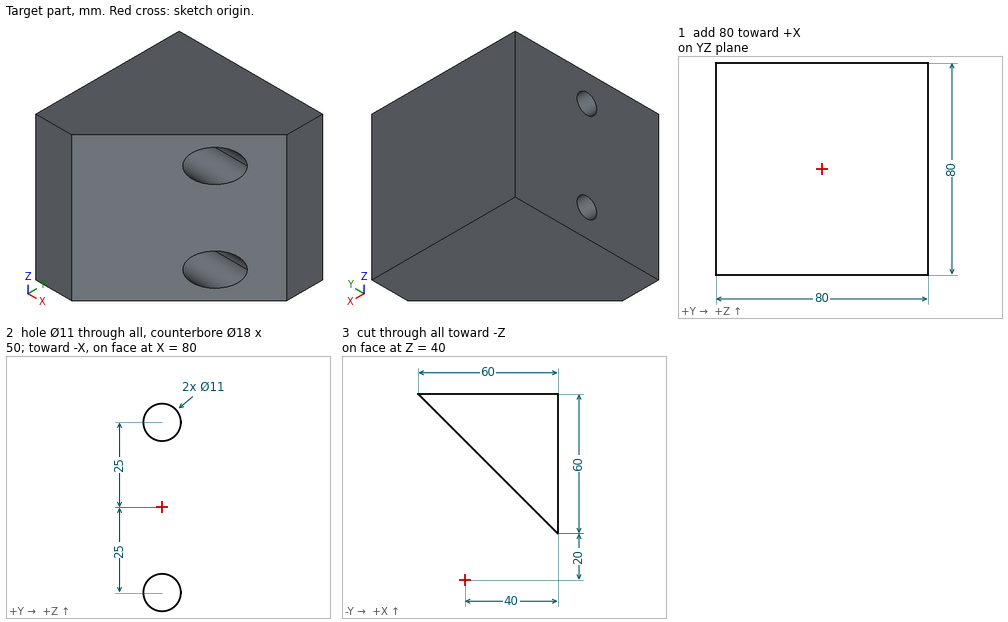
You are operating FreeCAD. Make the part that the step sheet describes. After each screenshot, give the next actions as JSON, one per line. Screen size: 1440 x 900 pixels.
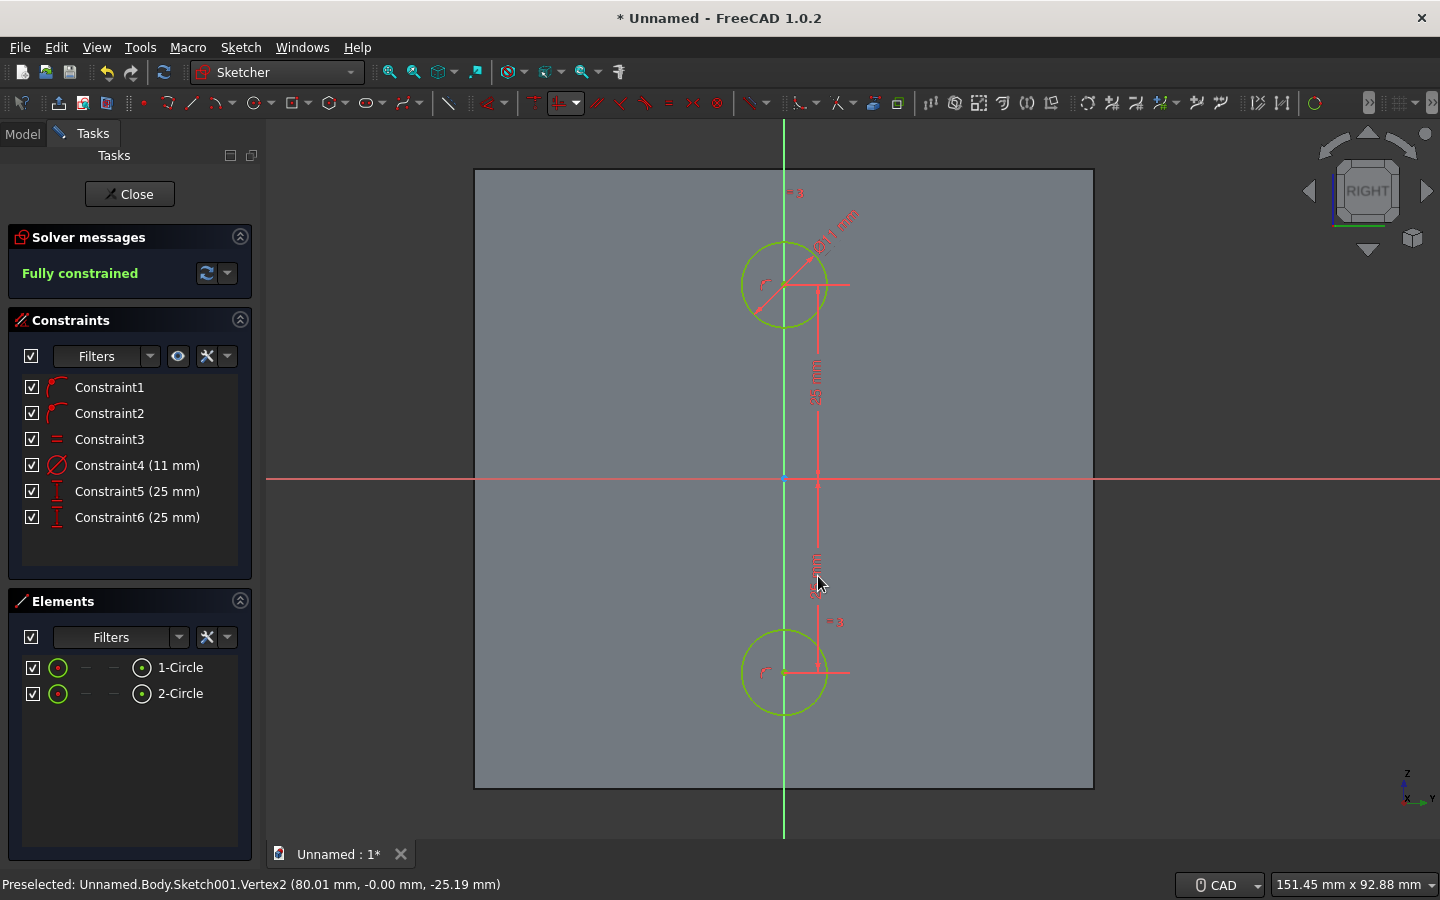
{"action": "left_click", "coordinate": [130, 194]}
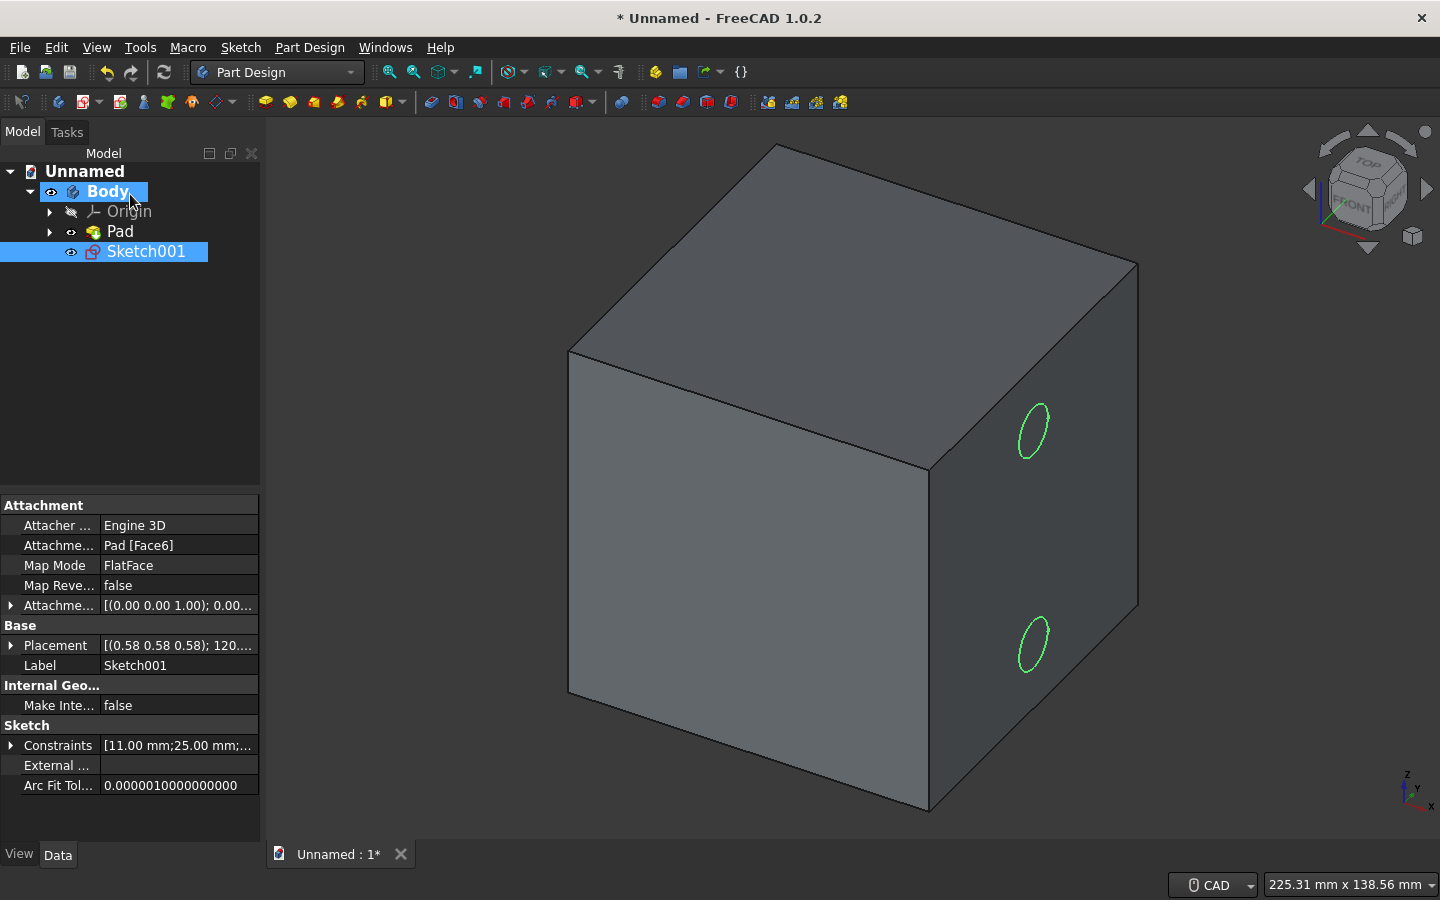
{"action": "left_click", "coordinate": [456, 102]}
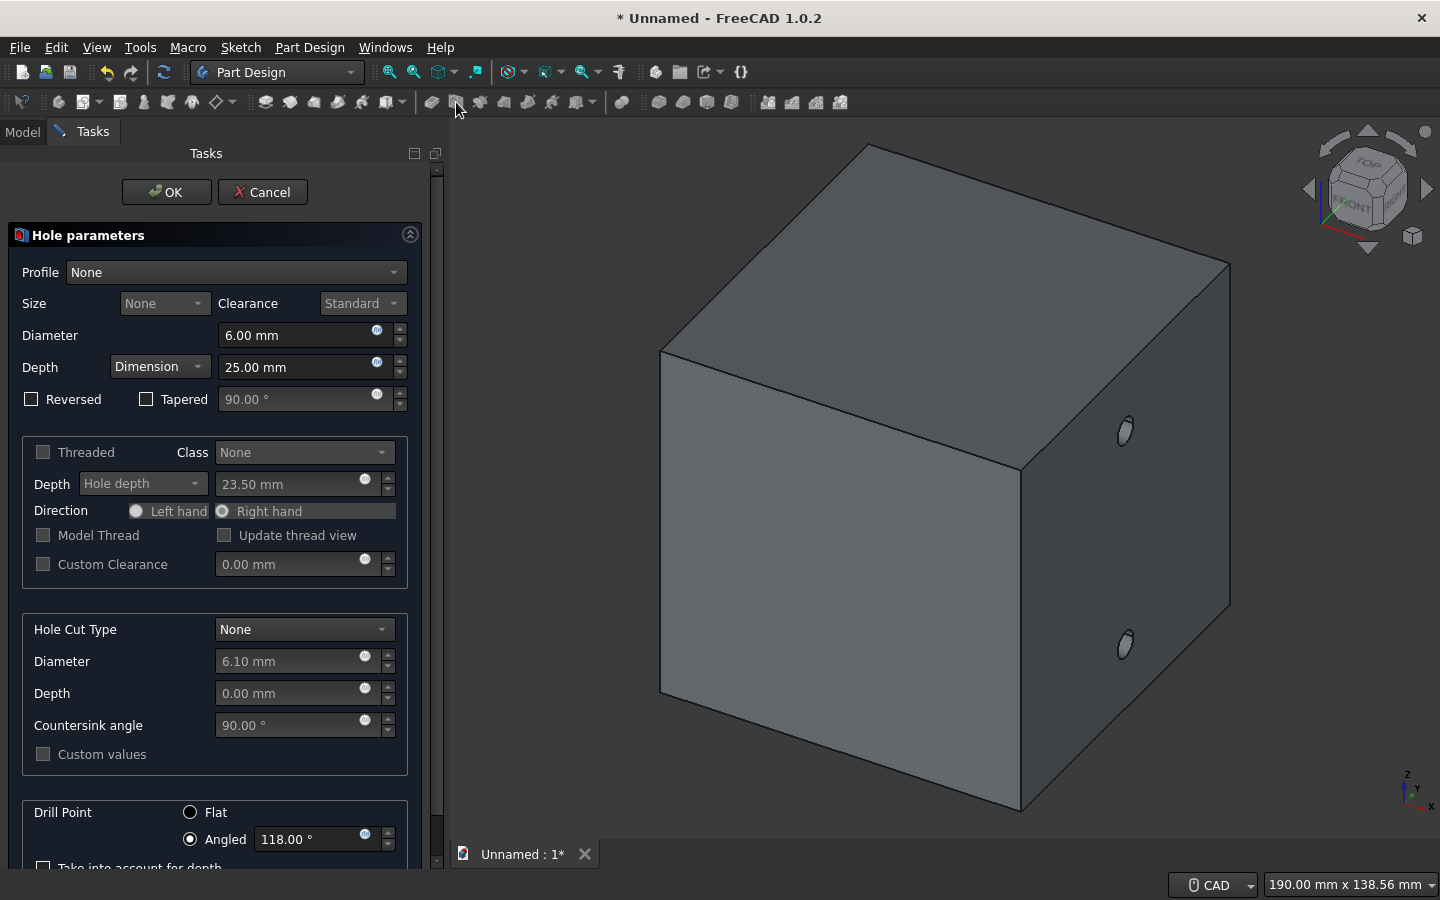
{"action": "triple_click", "coordinate": [305, 335]}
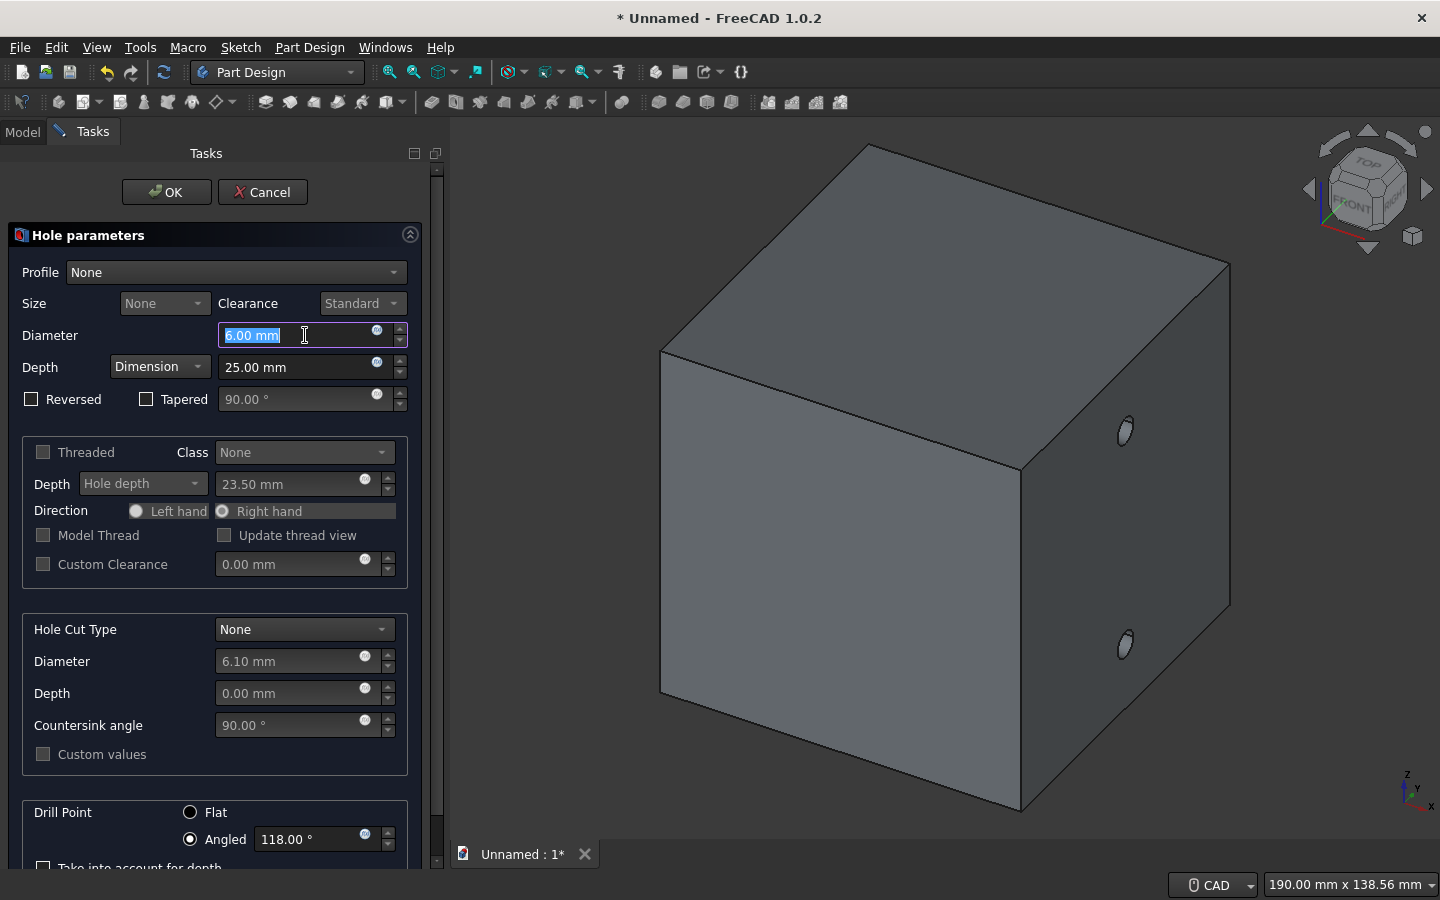
{"action": "type", "text": "11"}
{"action": "key", "text": "Tab"}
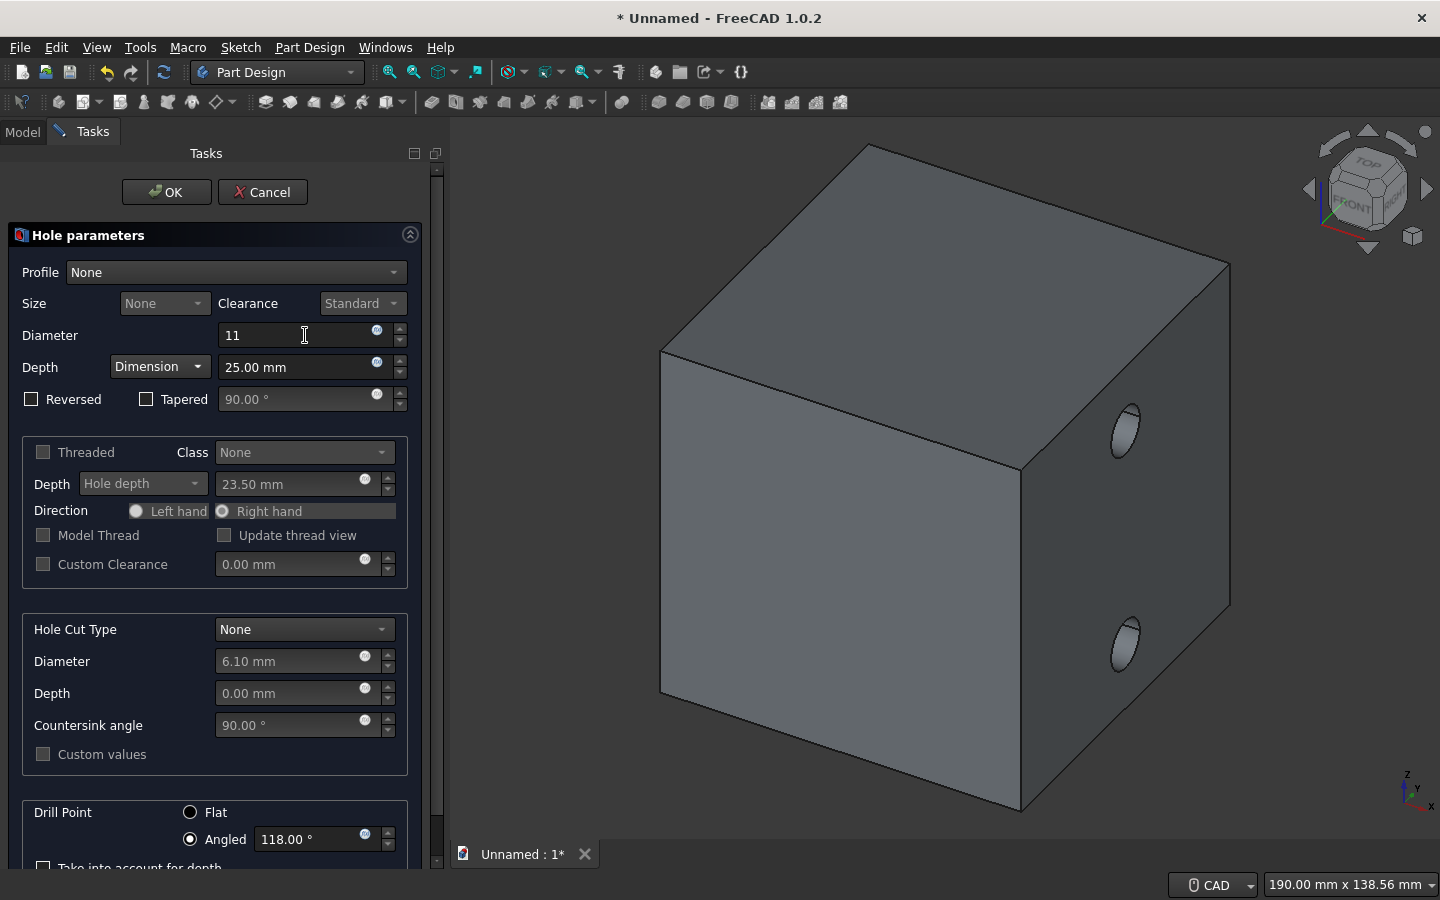
{"action": "left_click", "coordinate": [161, 366]}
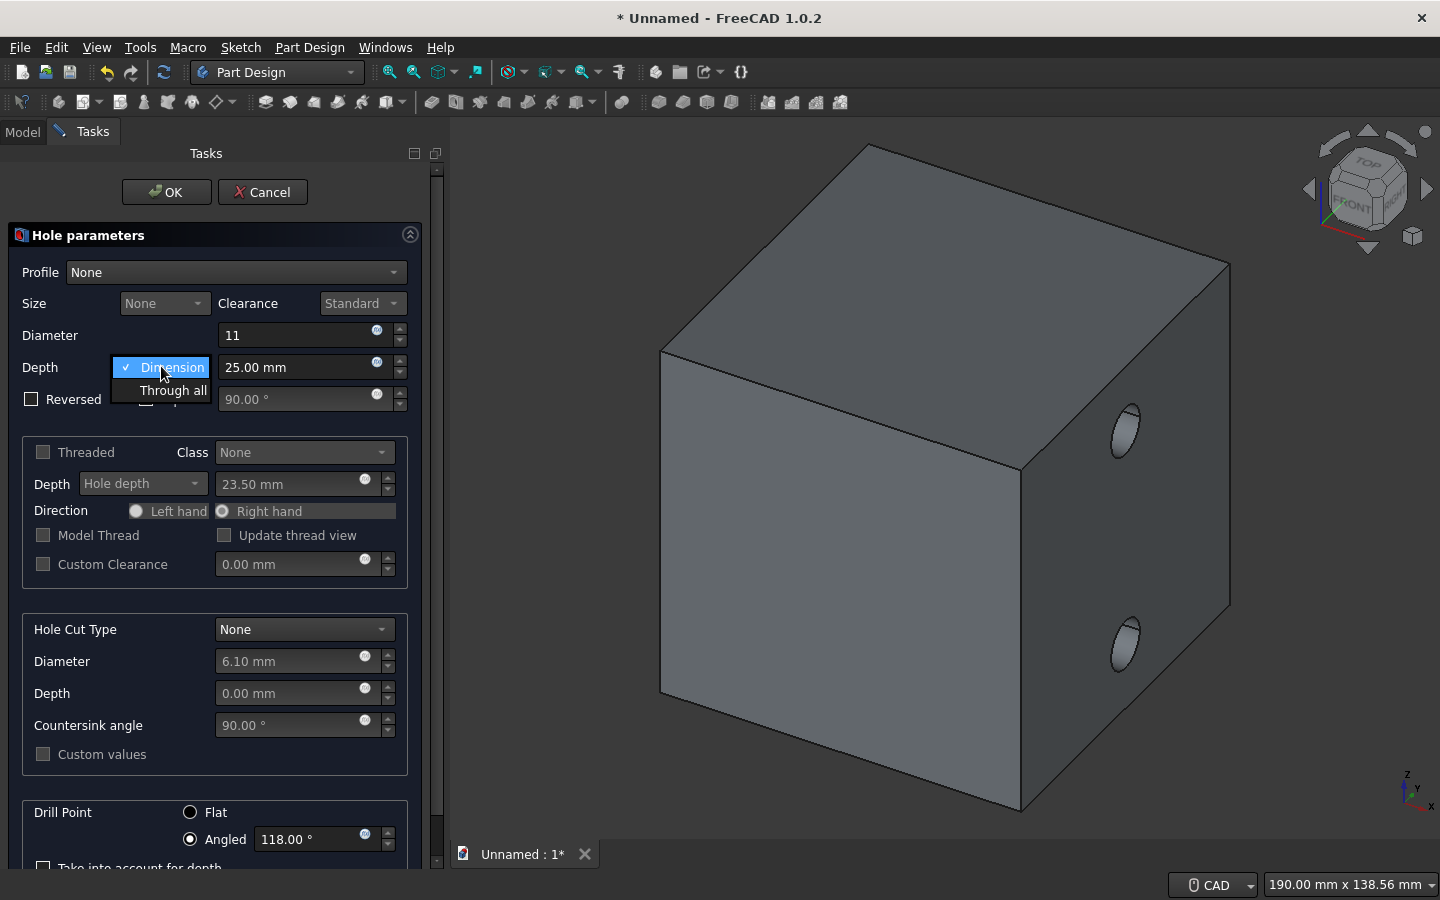
{"action": "left_click", "coordinate": [160, 390]}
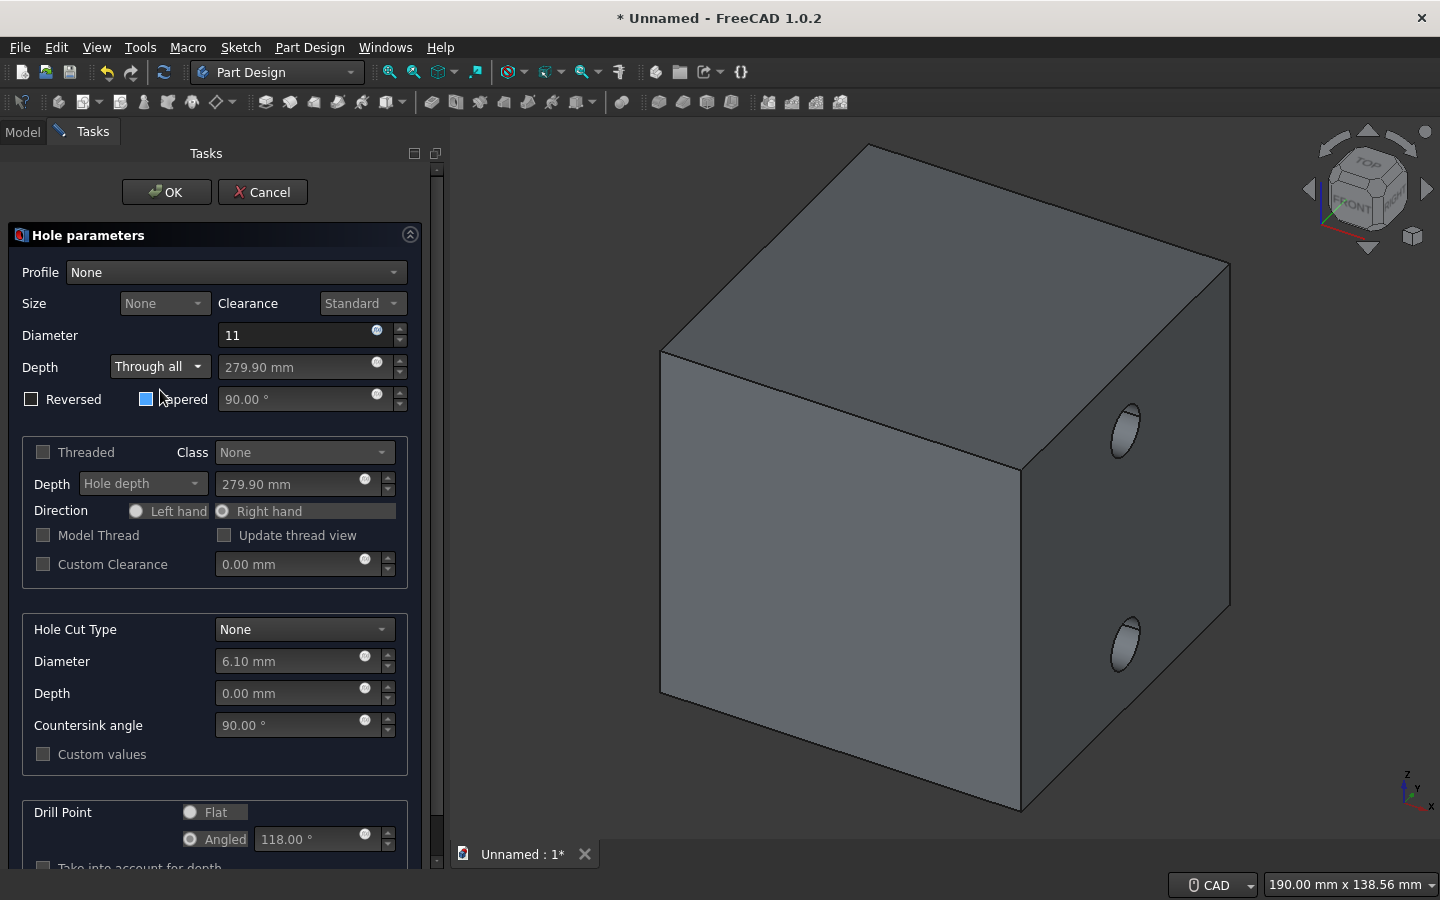
{"action": "left_click", "coordinate": [306, 630]}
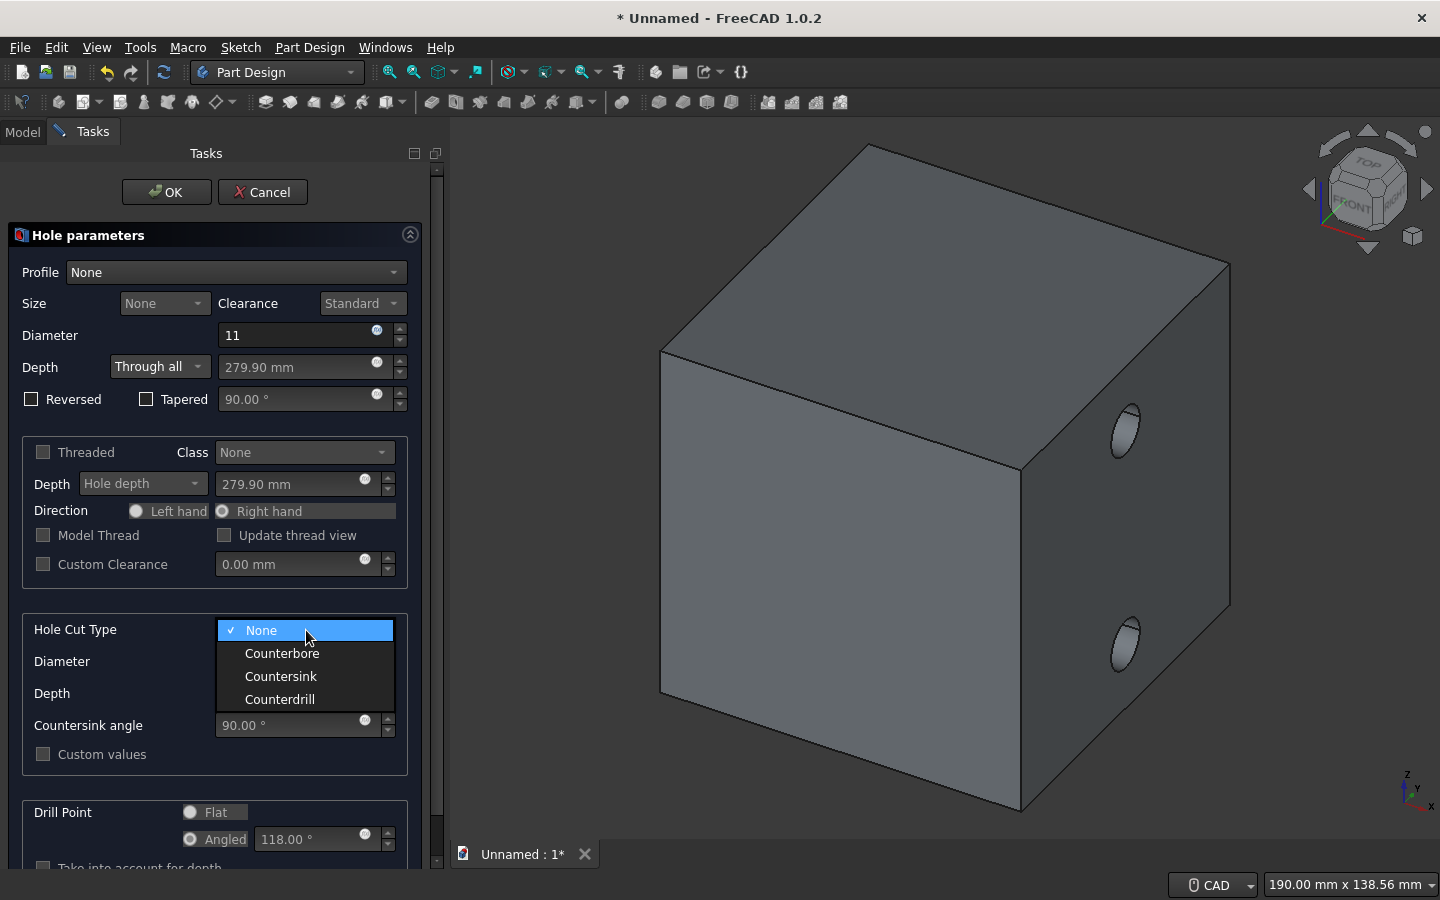
{"action": "left_click", "coordinate": [304, 654]}